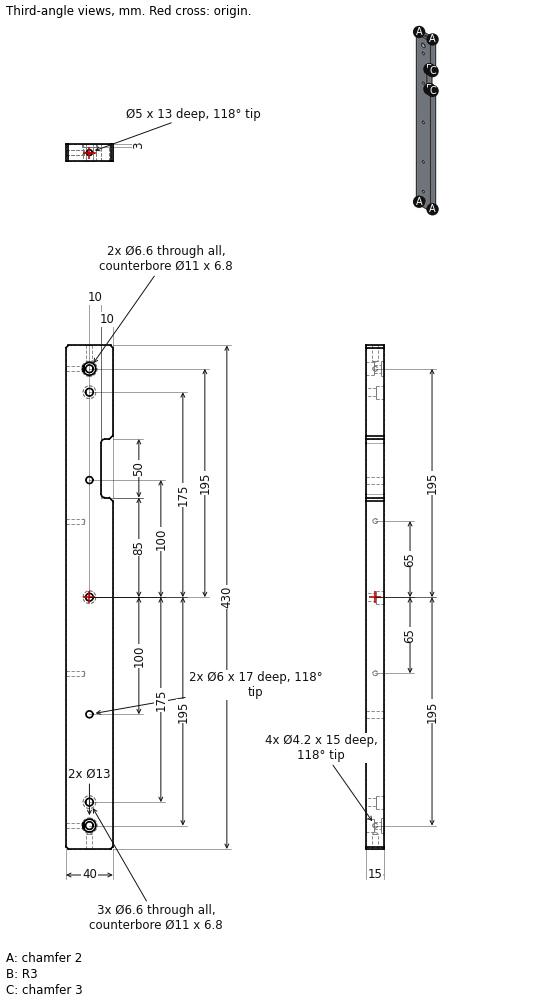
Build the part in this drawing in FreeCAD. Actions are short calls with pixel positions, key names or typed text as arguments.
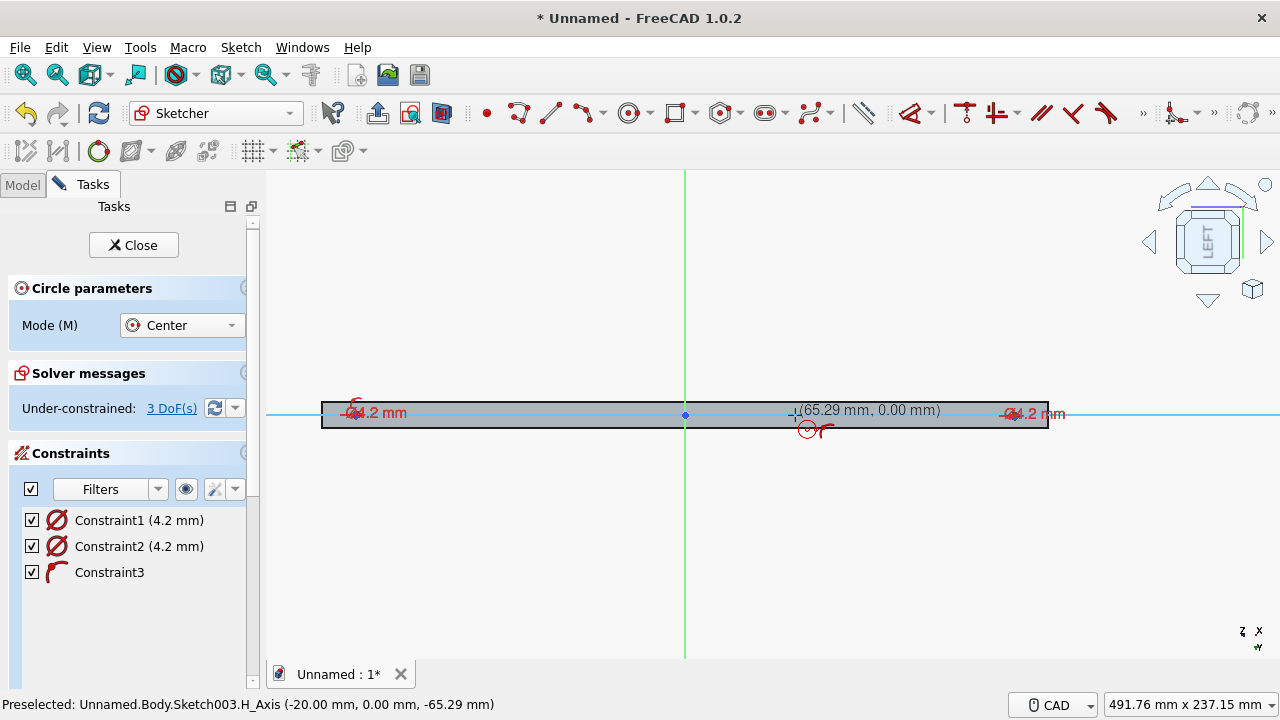
click(795, 415)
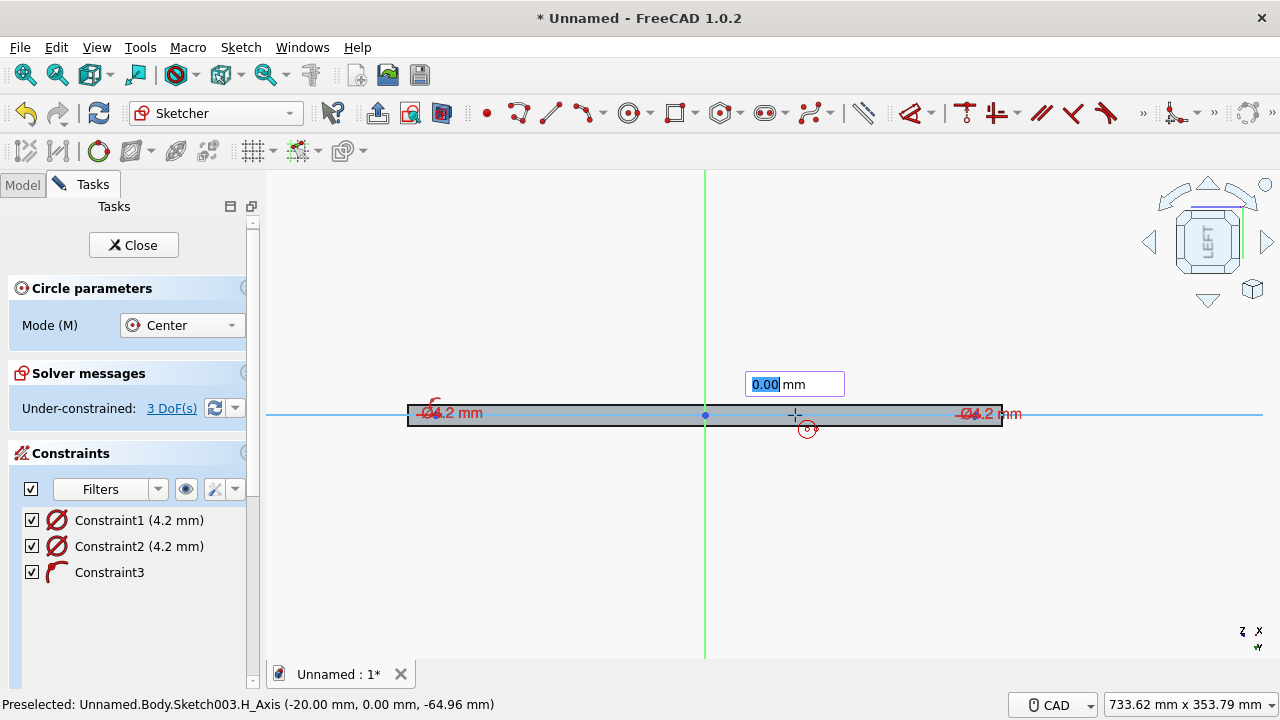
scroll(794, 418, up, 9)
move(792, 415)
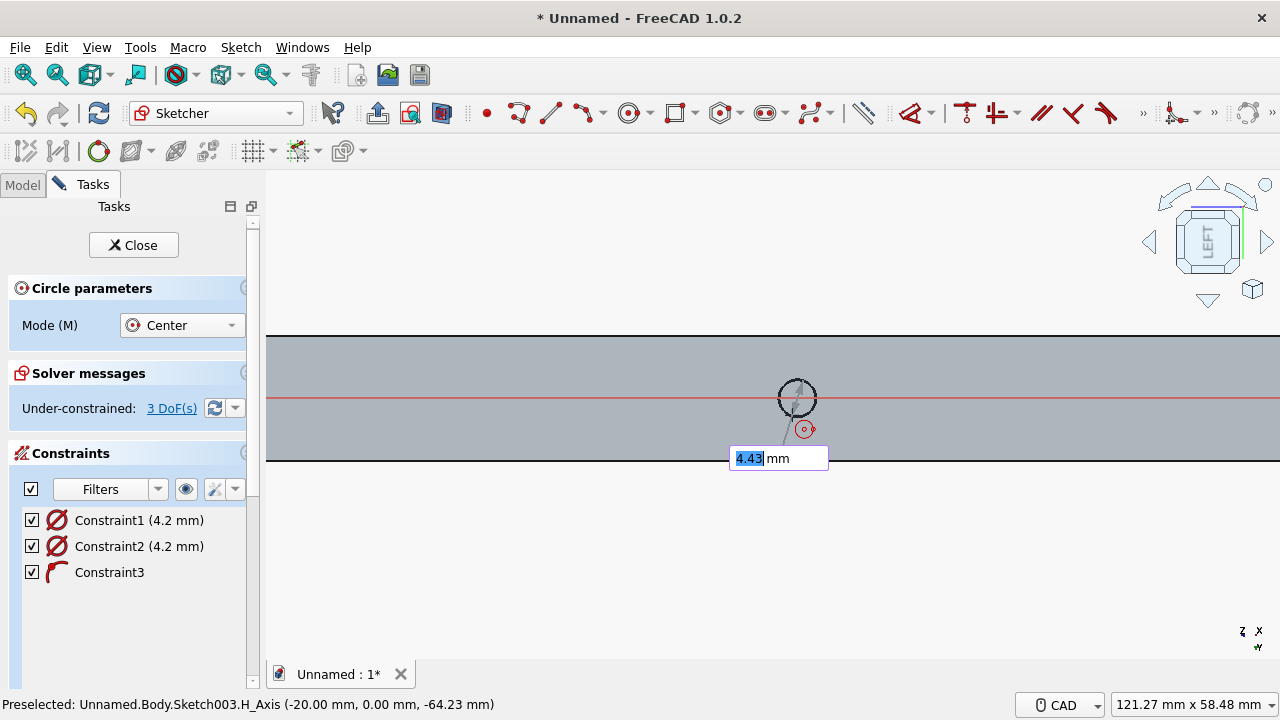
text(4.2)
key(Return)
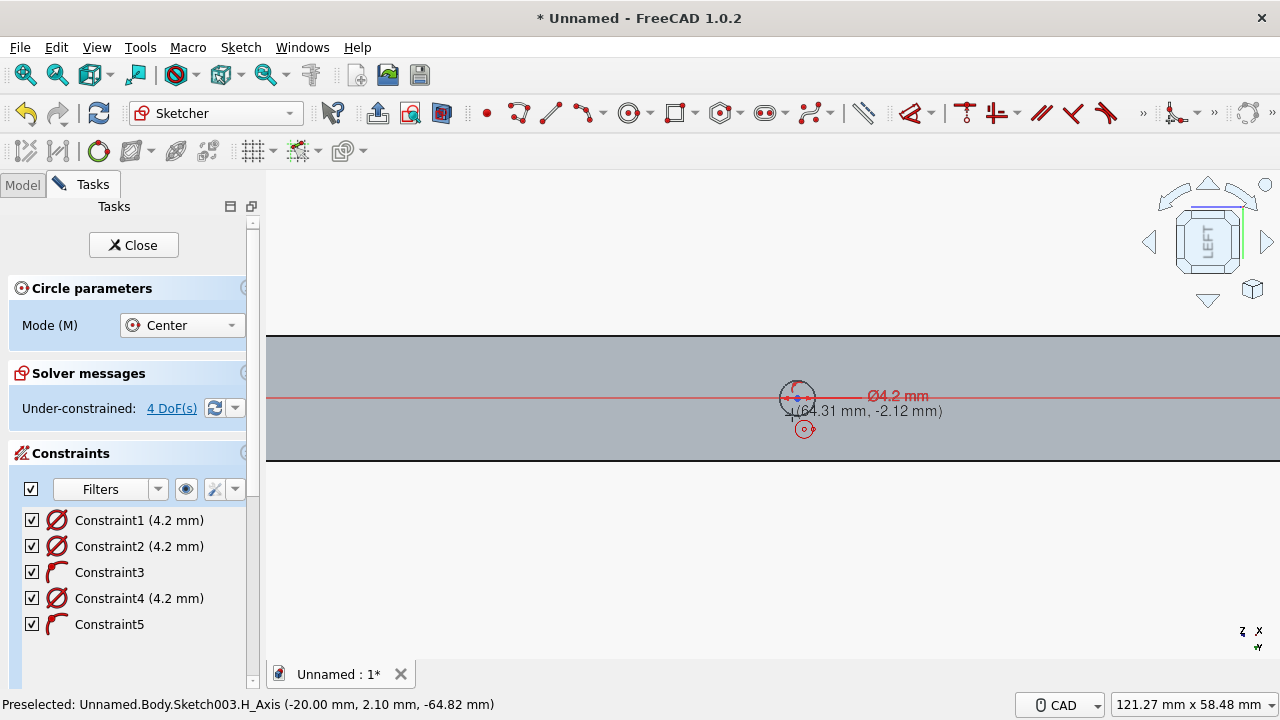
scroll(794, 418, down, 9)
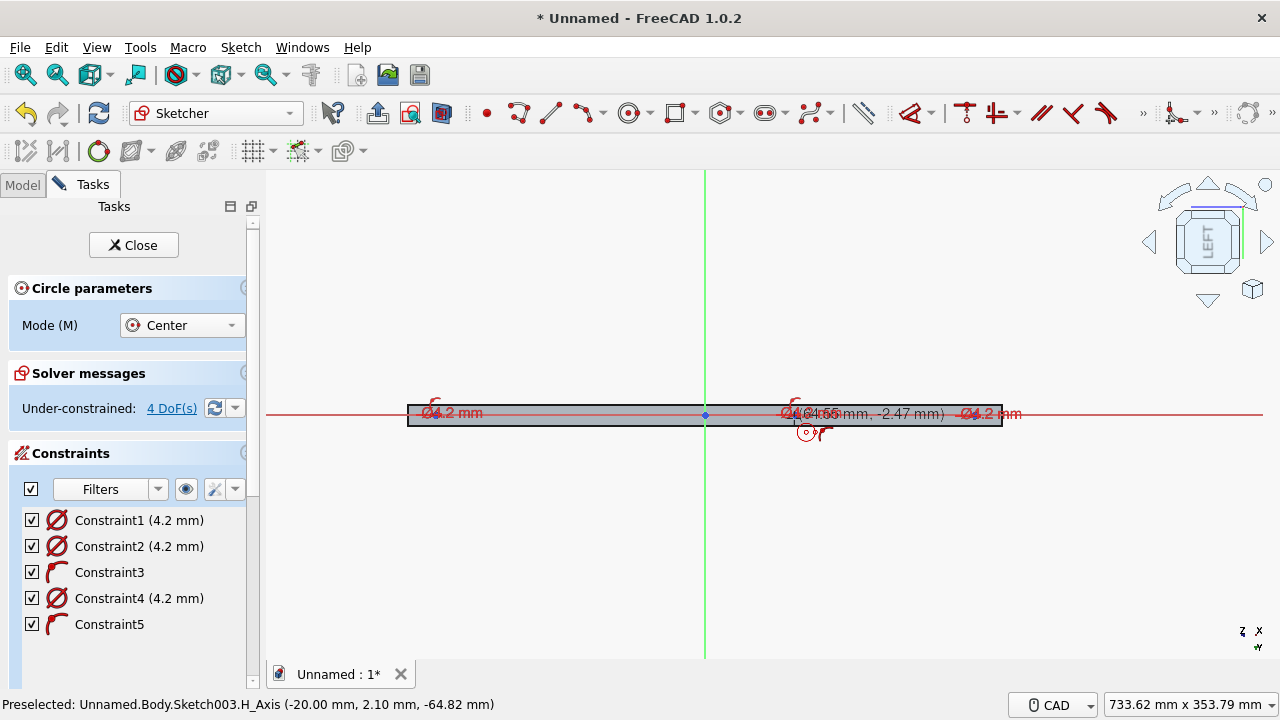
scroll(615, 415, up, 11)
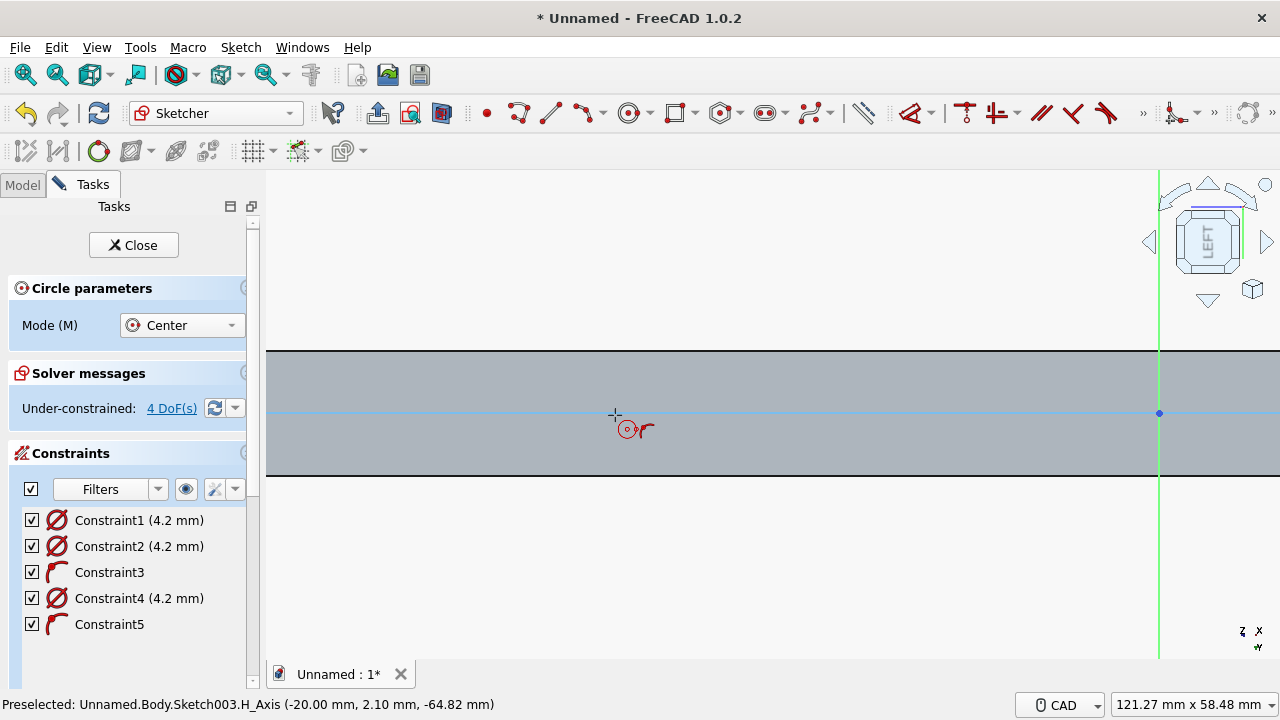
scroll(615, 415, down, 11)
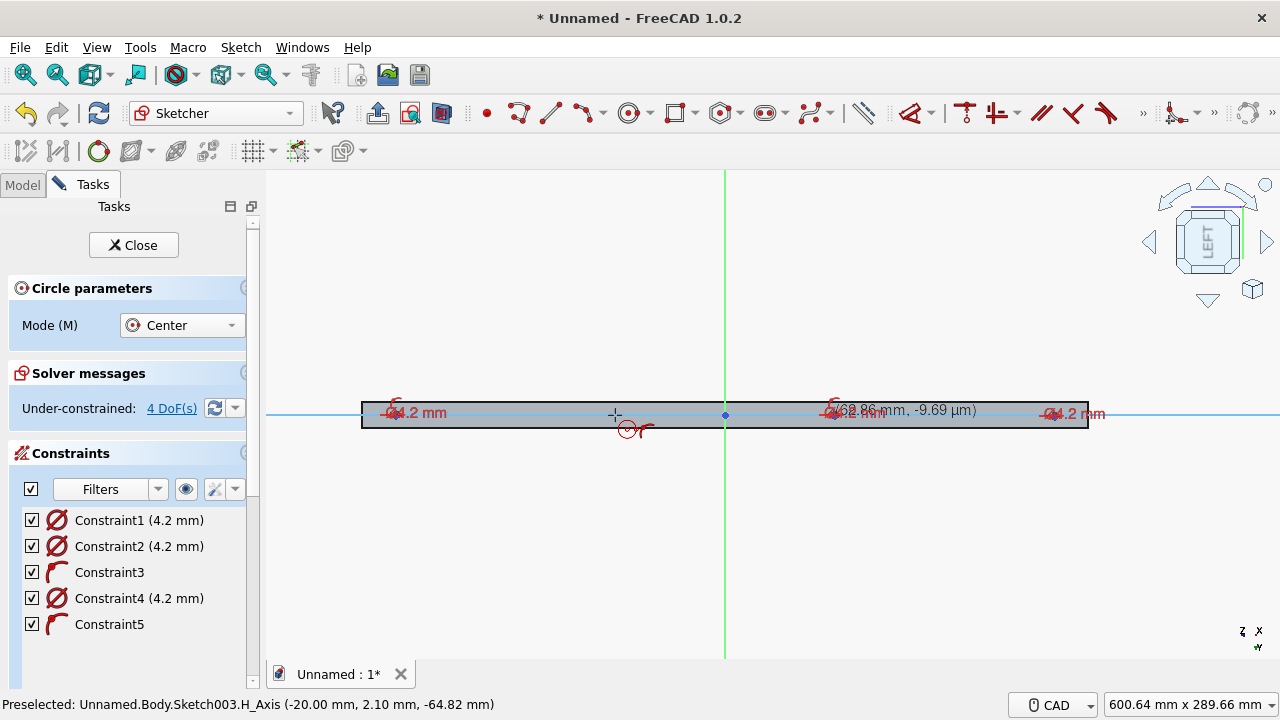
click(615, 415)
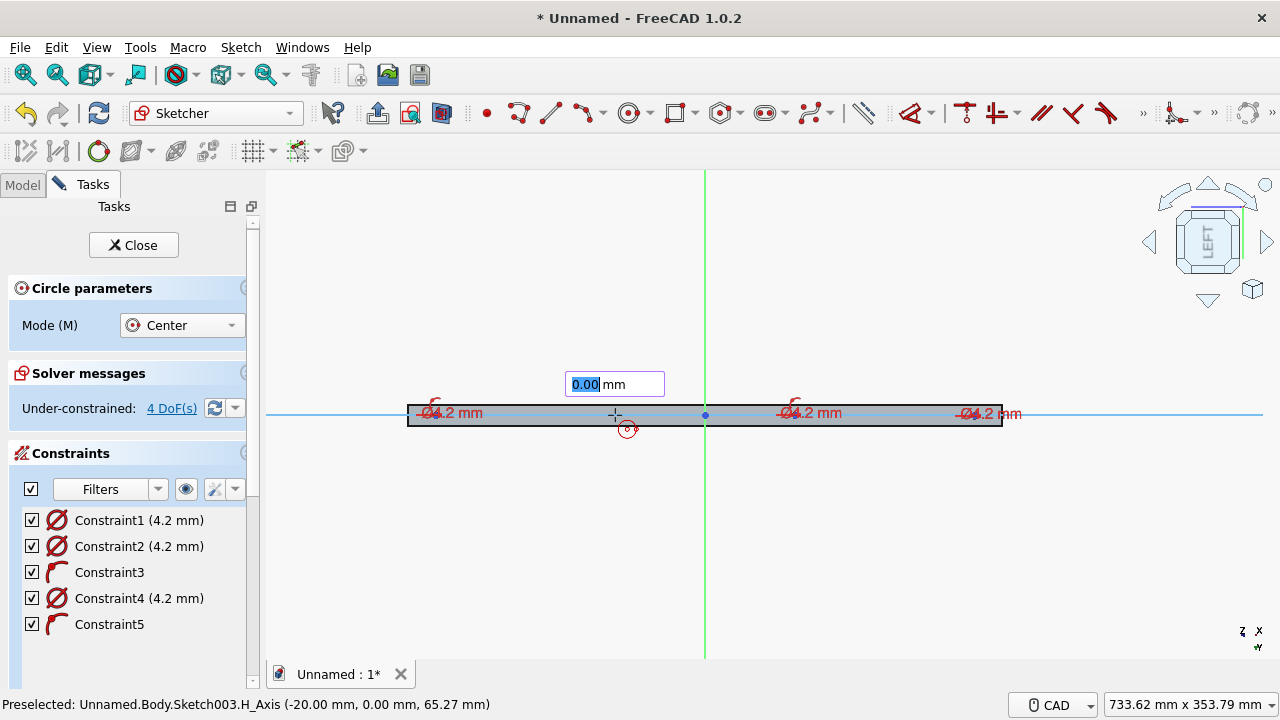
scroll(614, 418, up, 9)
move(615, 415)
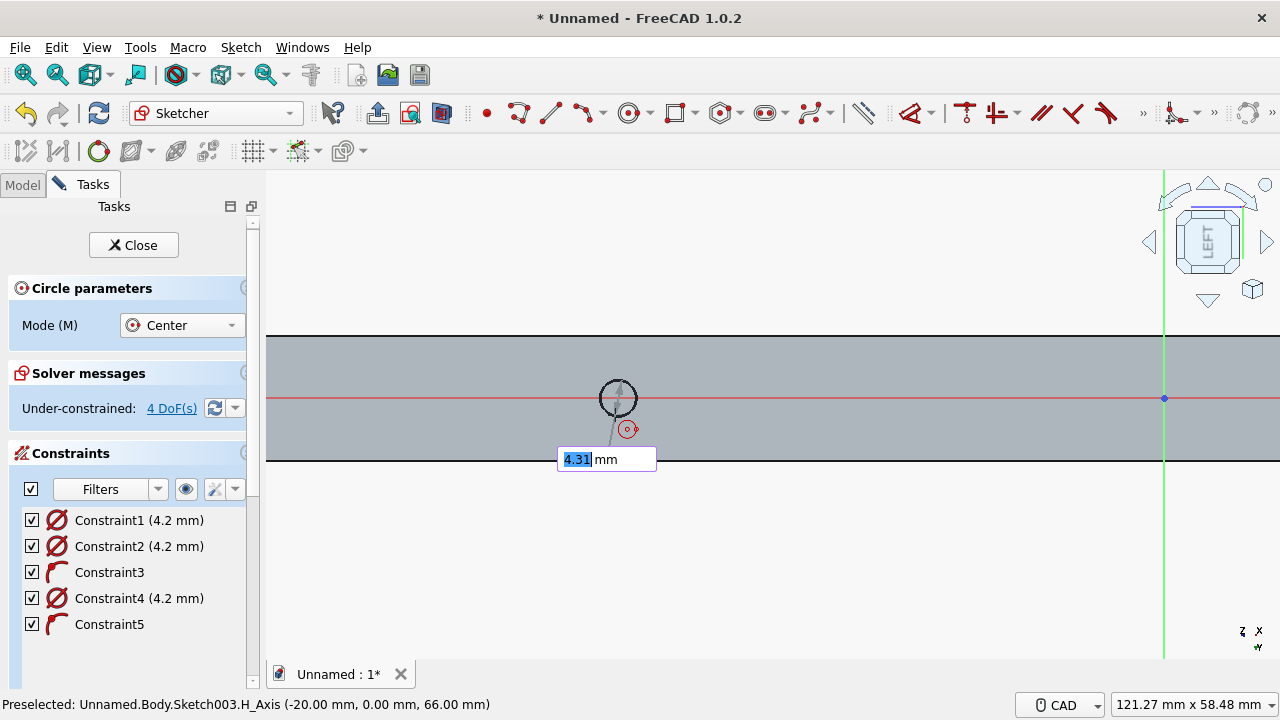
text(4.2)
key(Return)
key(Escape)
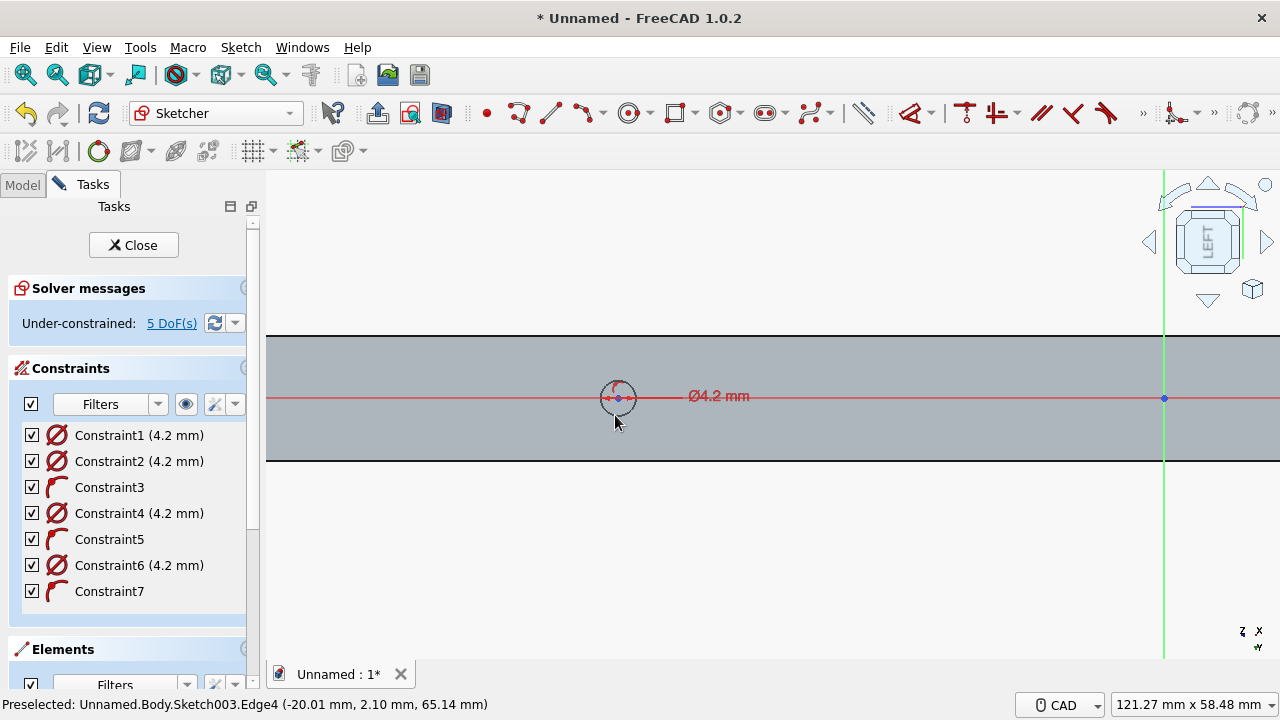
scroll(613, 418, down, 9)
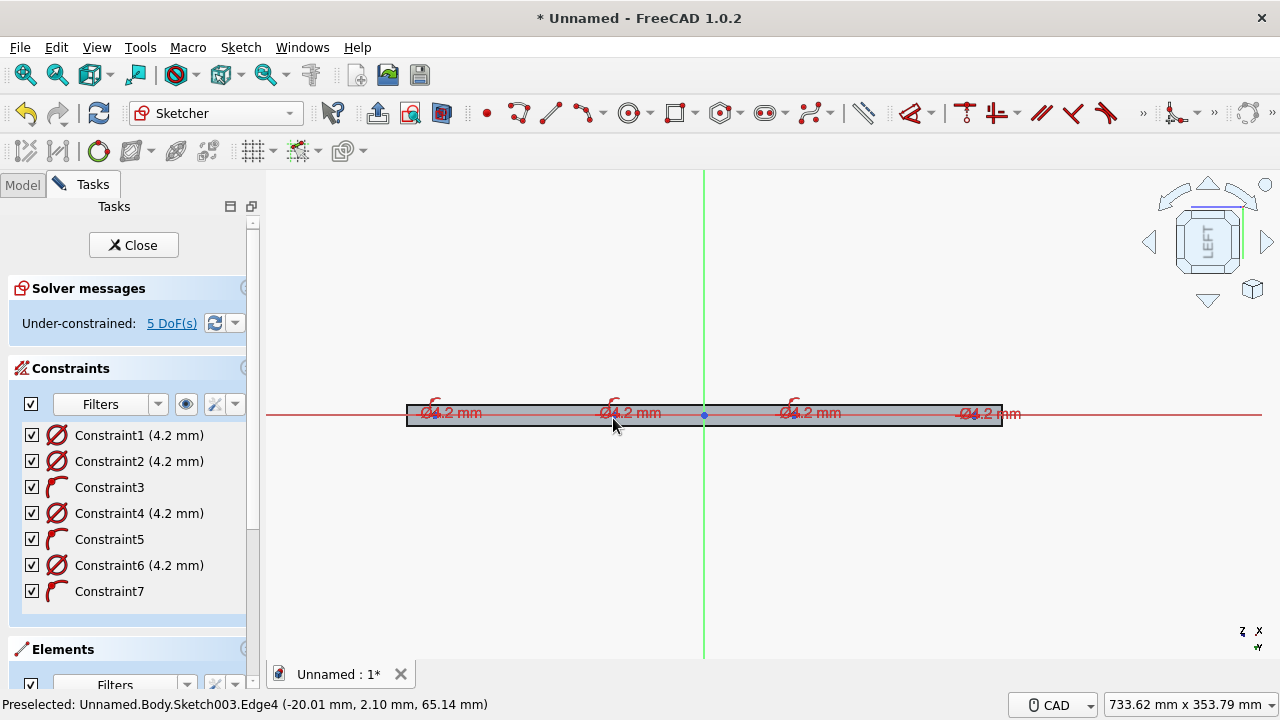
click(974, 416)